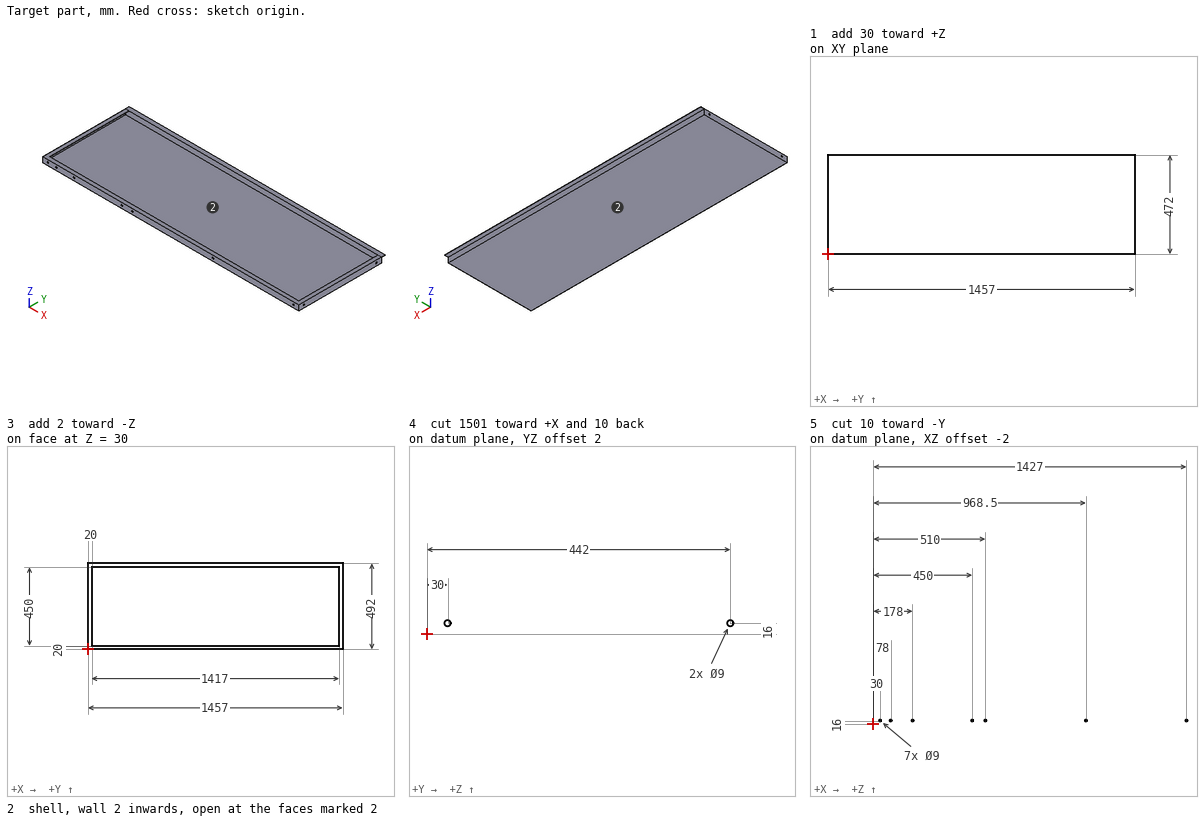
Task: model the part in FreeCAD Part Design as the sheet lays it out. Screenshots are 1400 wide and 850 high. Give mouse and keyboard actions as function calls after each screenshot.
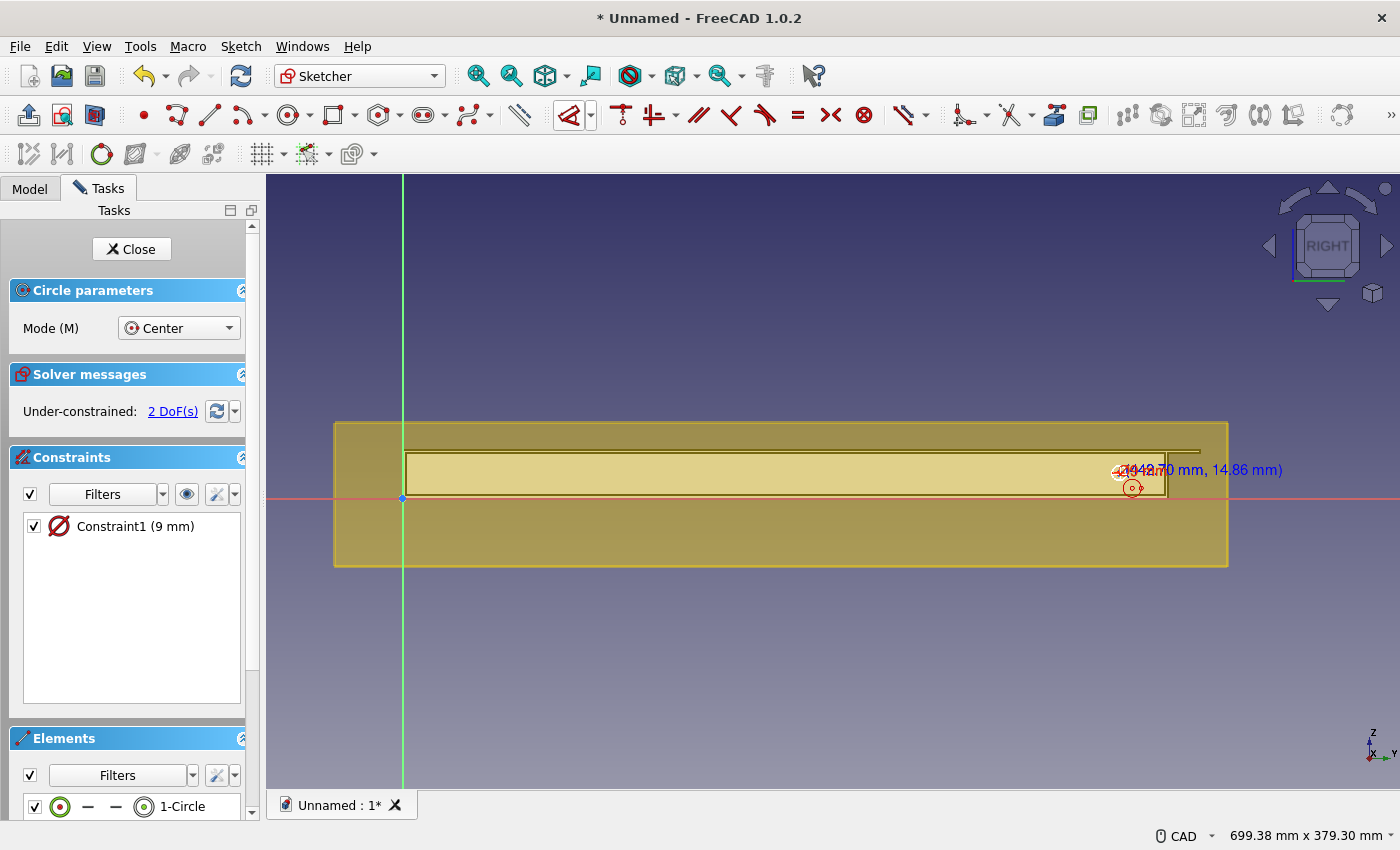
scroll(451, 473, up, 6)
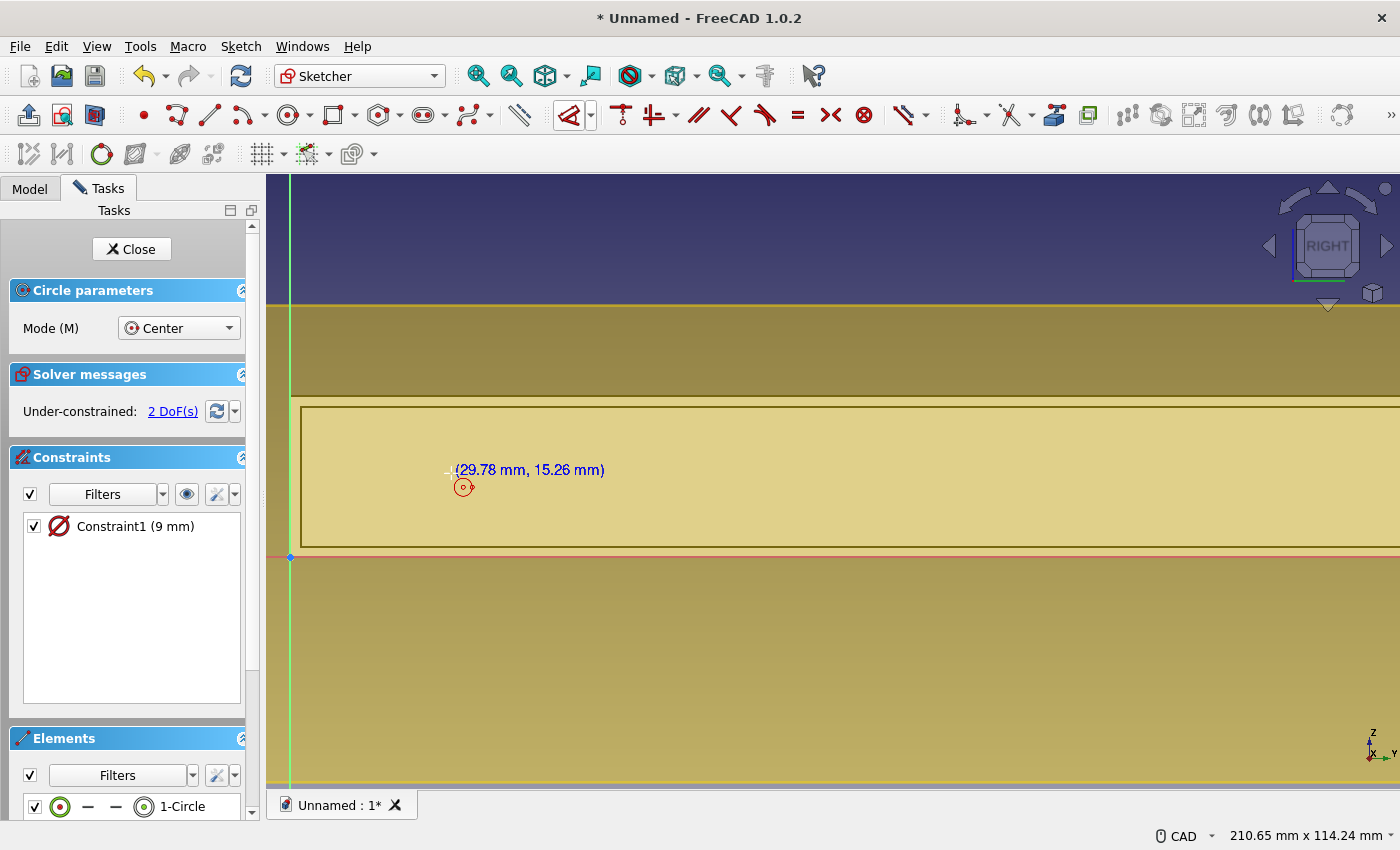
click(452, 471)
move(469, 454)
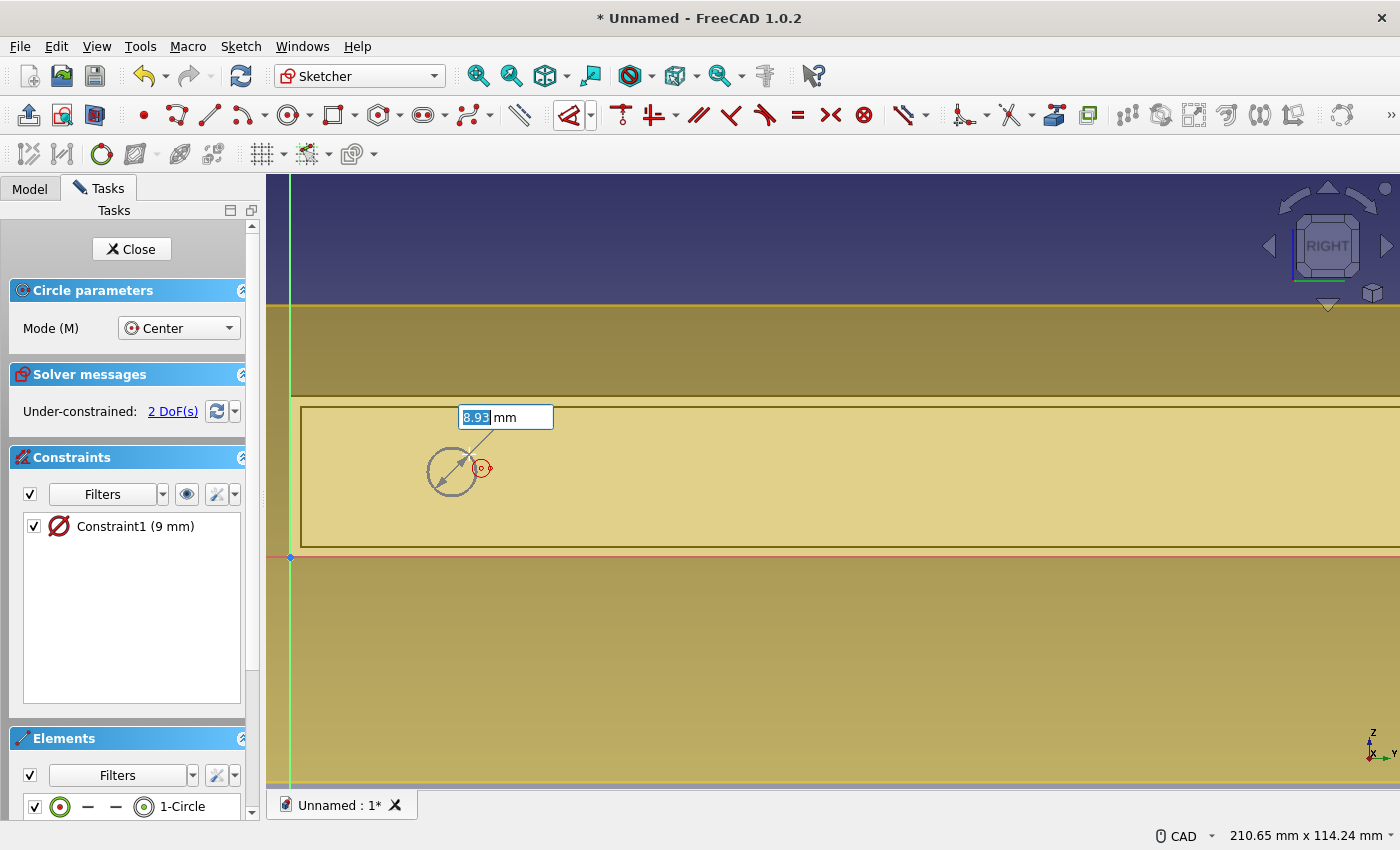
text(9)
key(Return)
key(Escape)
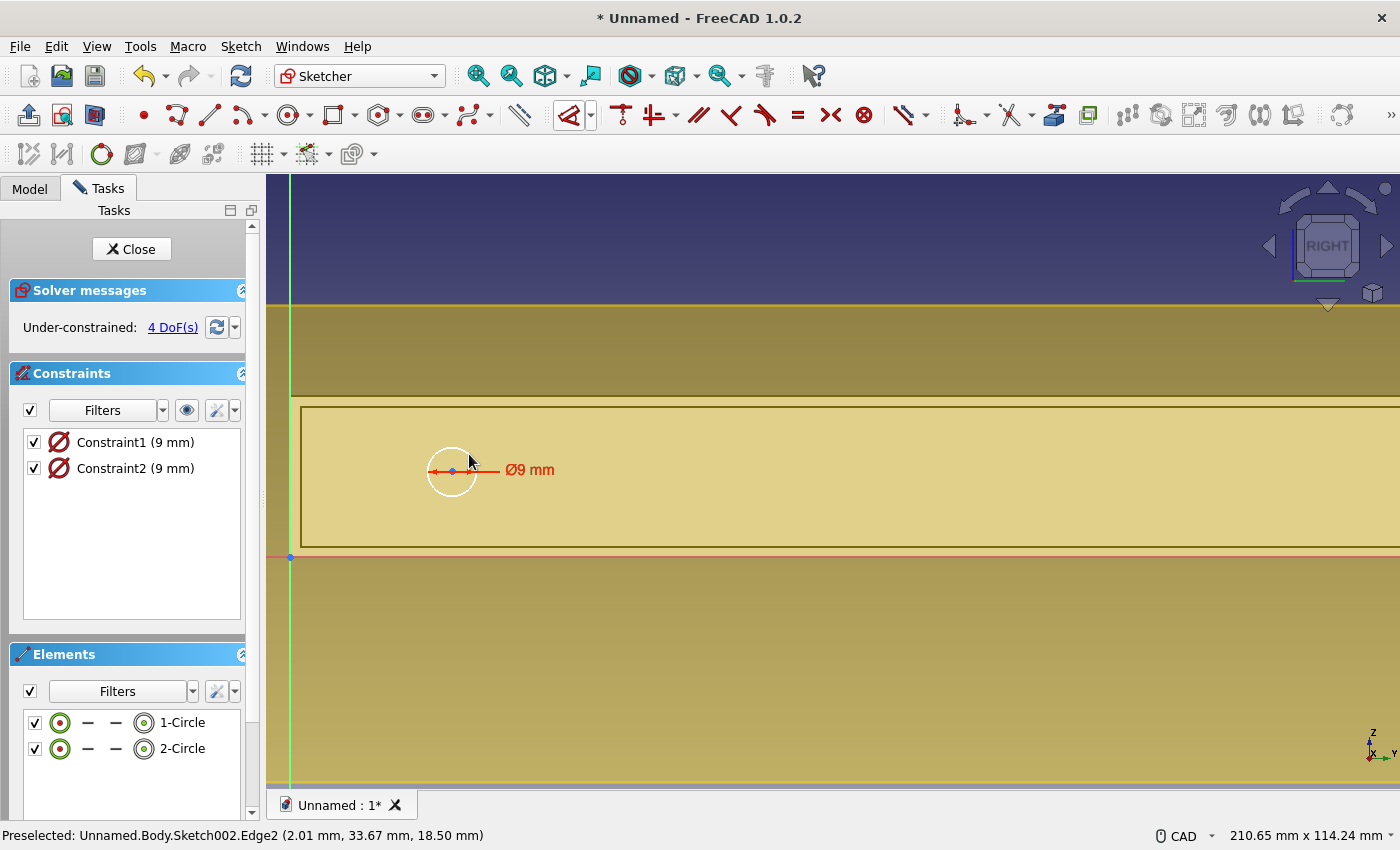
scroll(451, 473, down, 6)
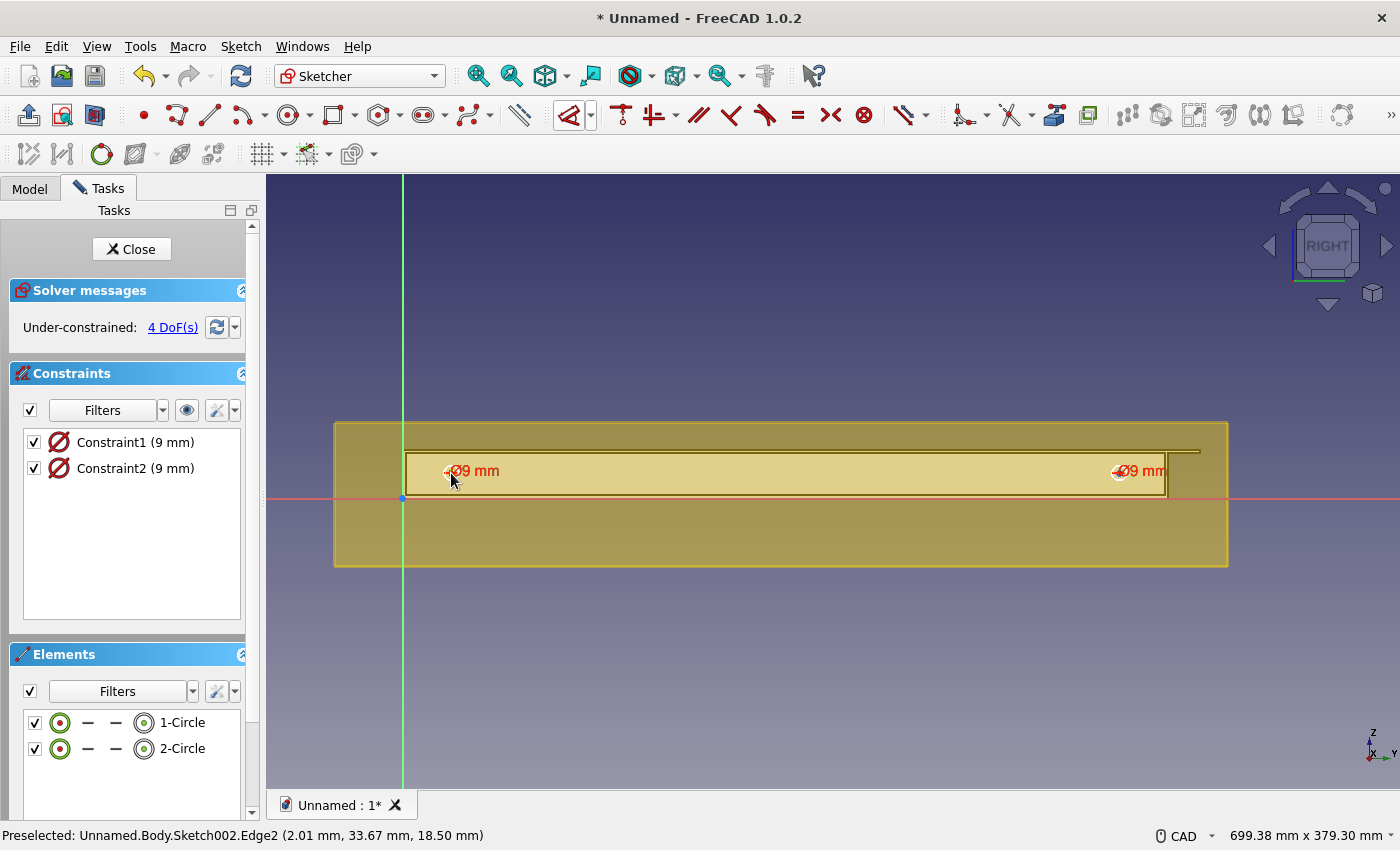
click(1119, 473)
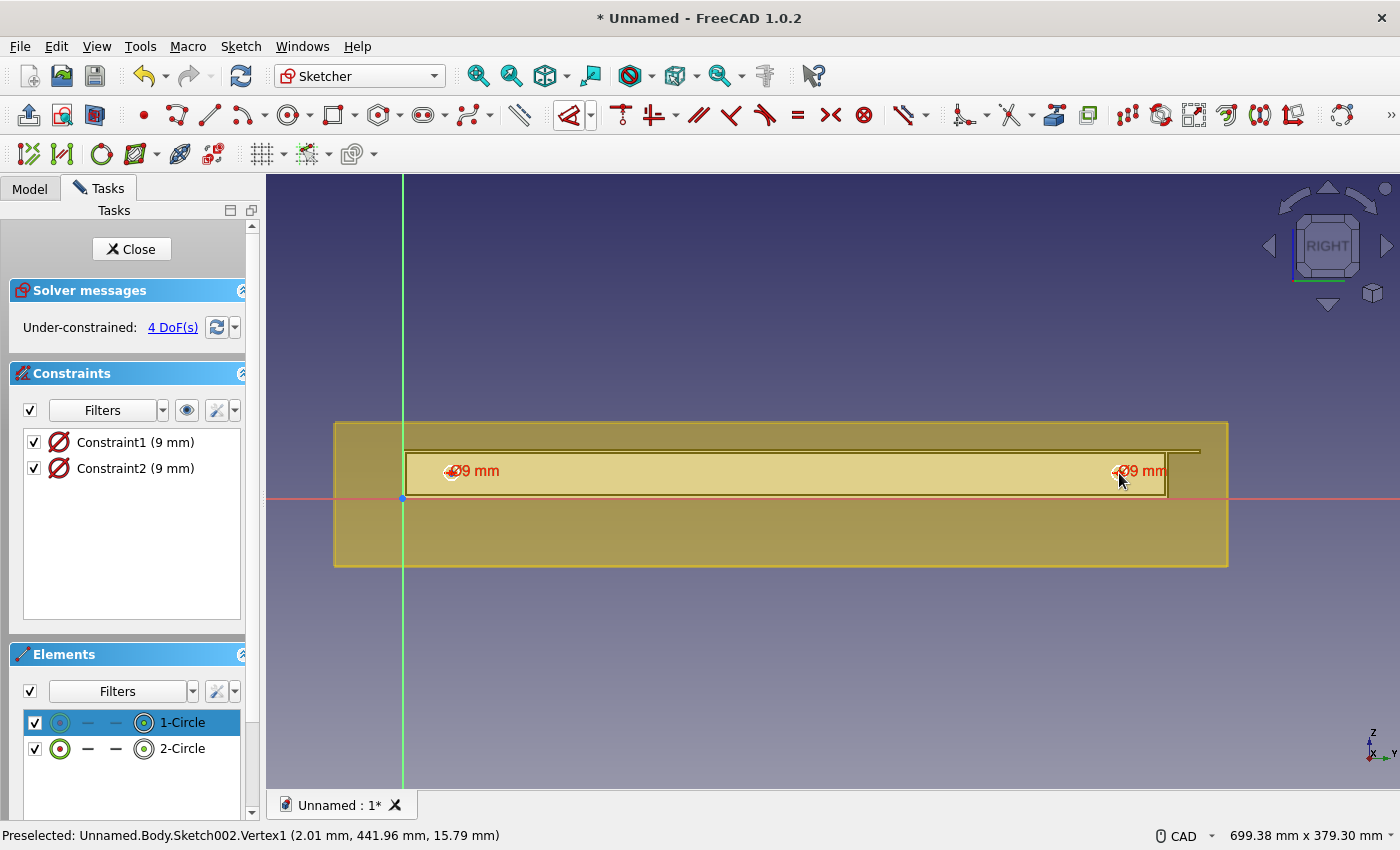
click(451, 473)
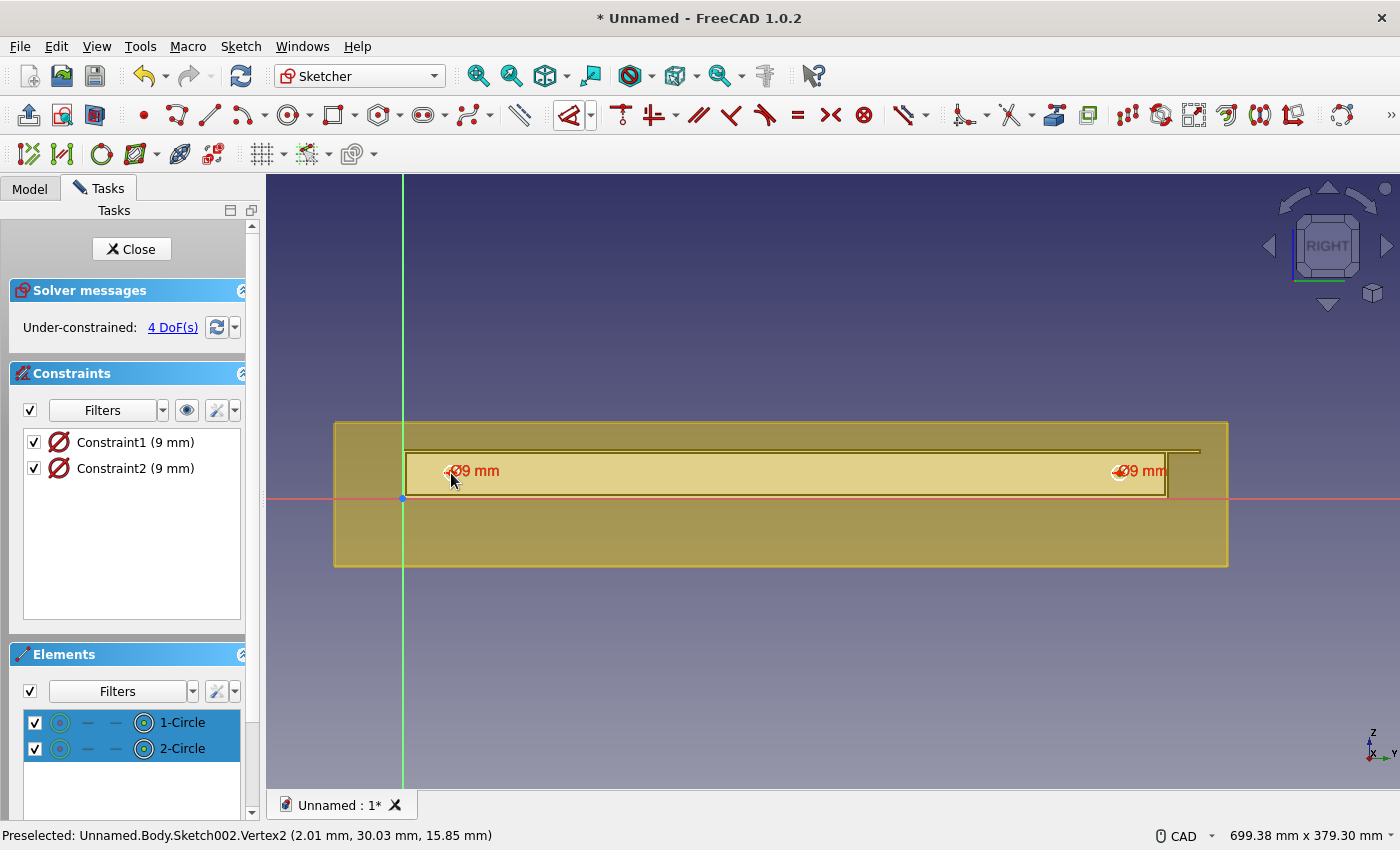
key(h)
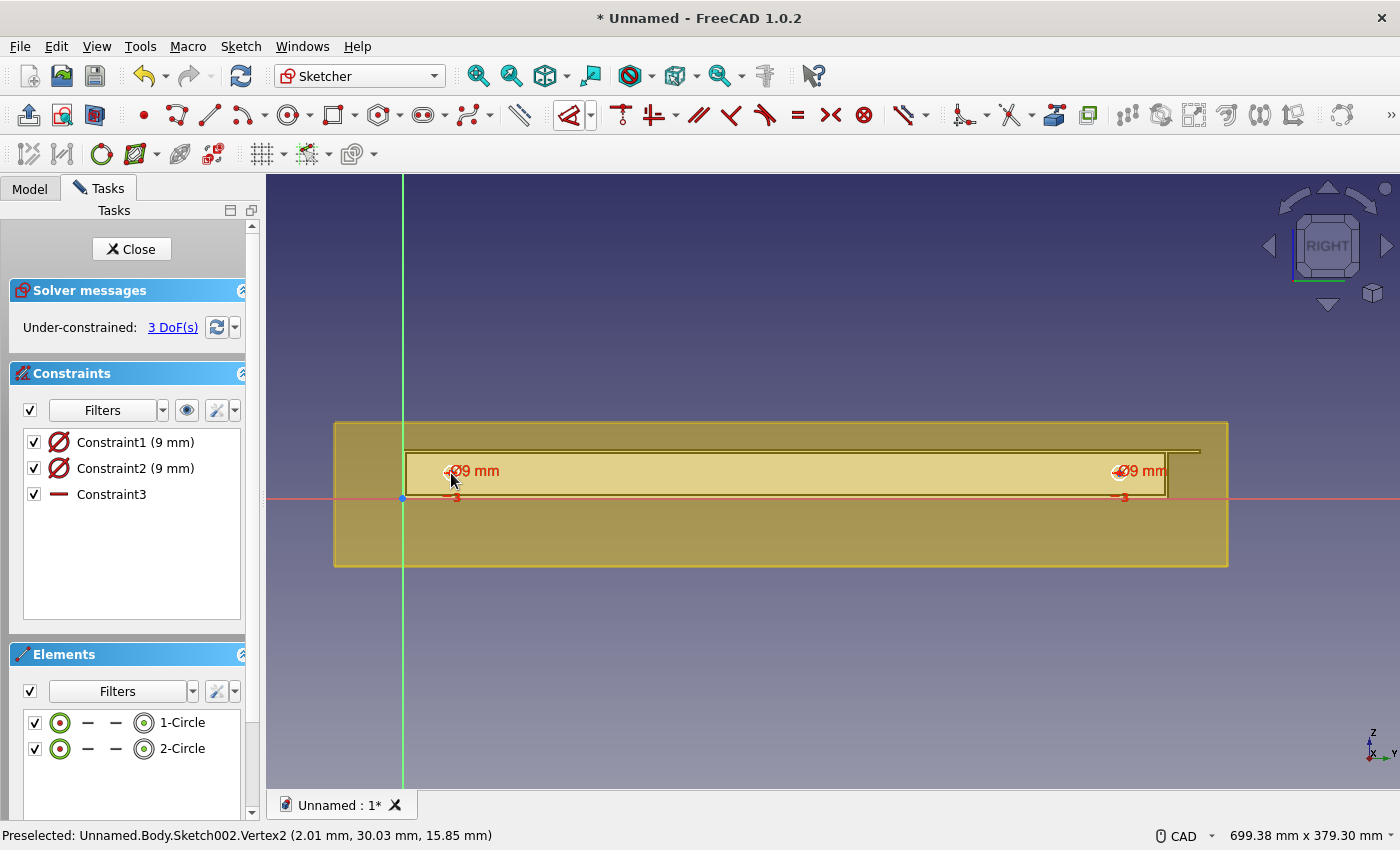
scroll(1119, 473, up, 3)